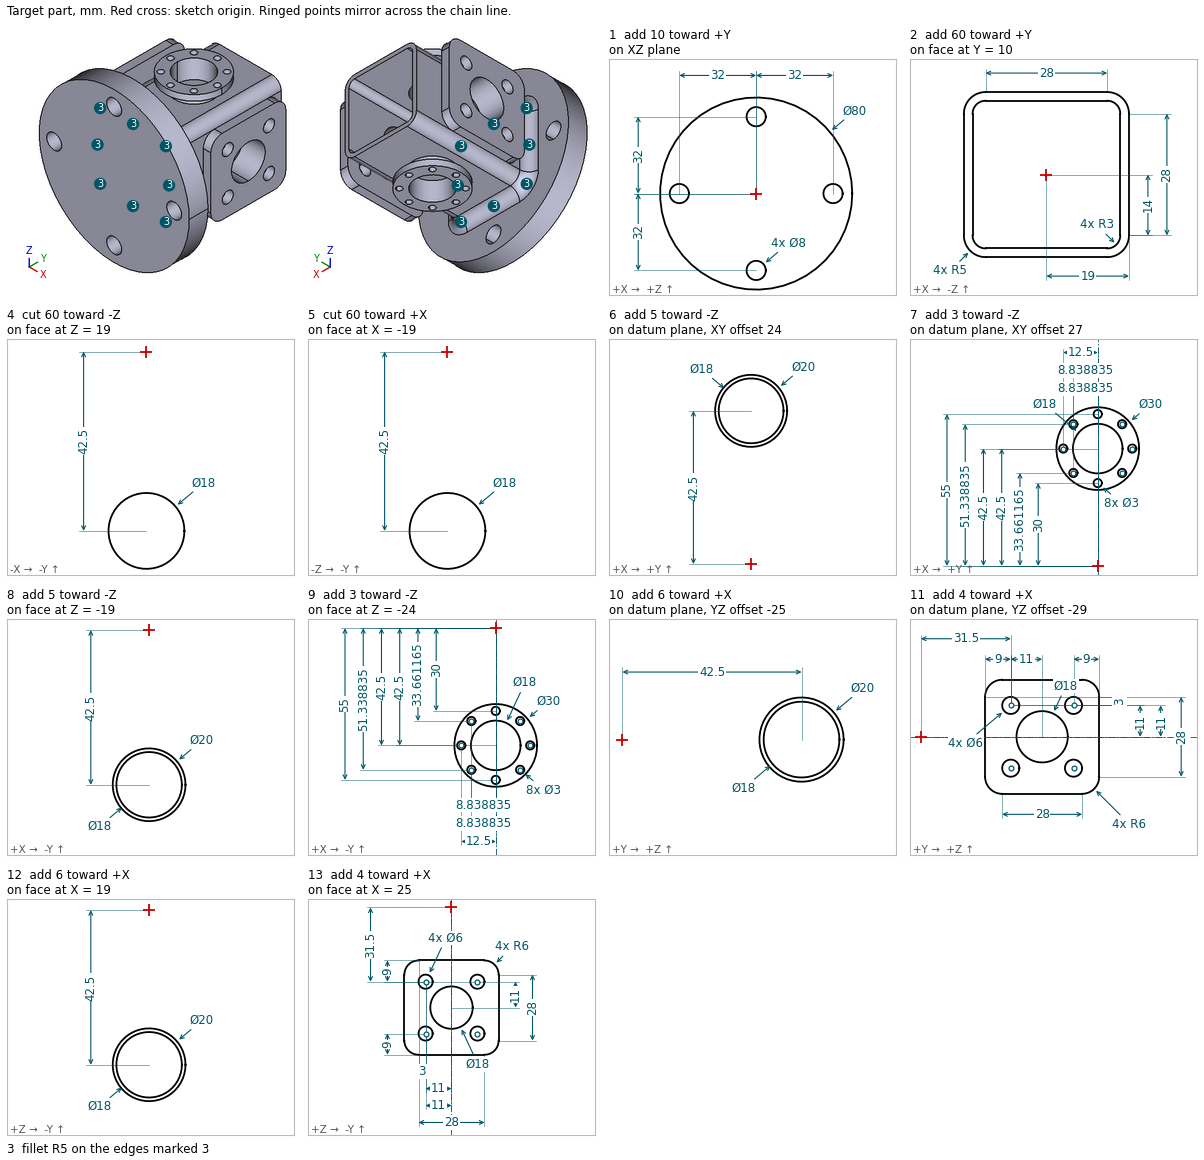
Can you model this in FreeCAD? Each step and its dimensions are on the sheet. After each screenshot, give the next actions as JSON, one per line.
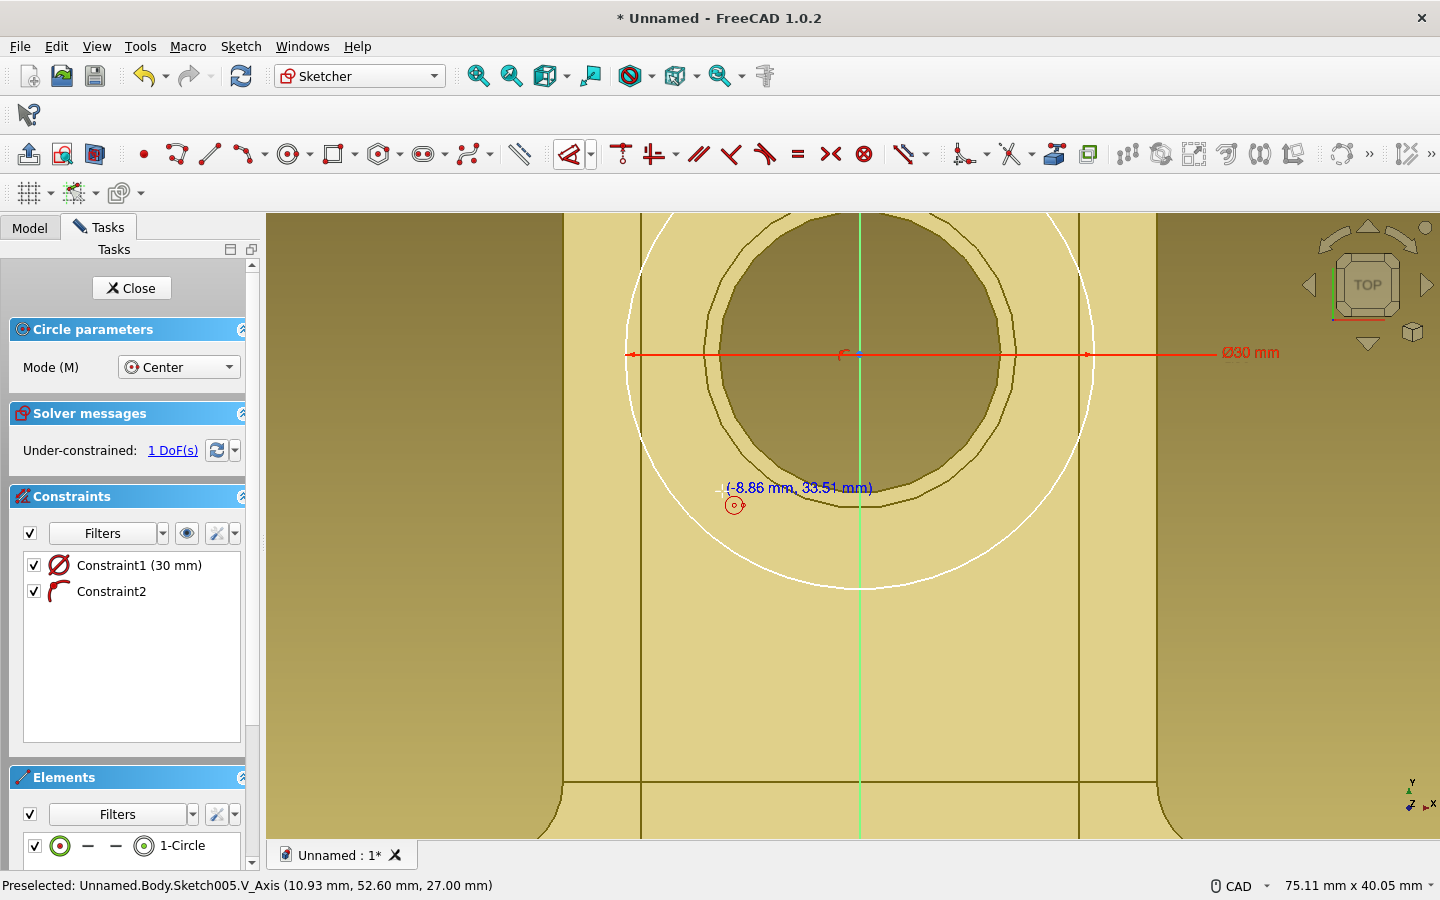
{"action": "left_click", "coordinate": [722, 490]}
{"action": "mouse_move", "coordinate": [738, 474]}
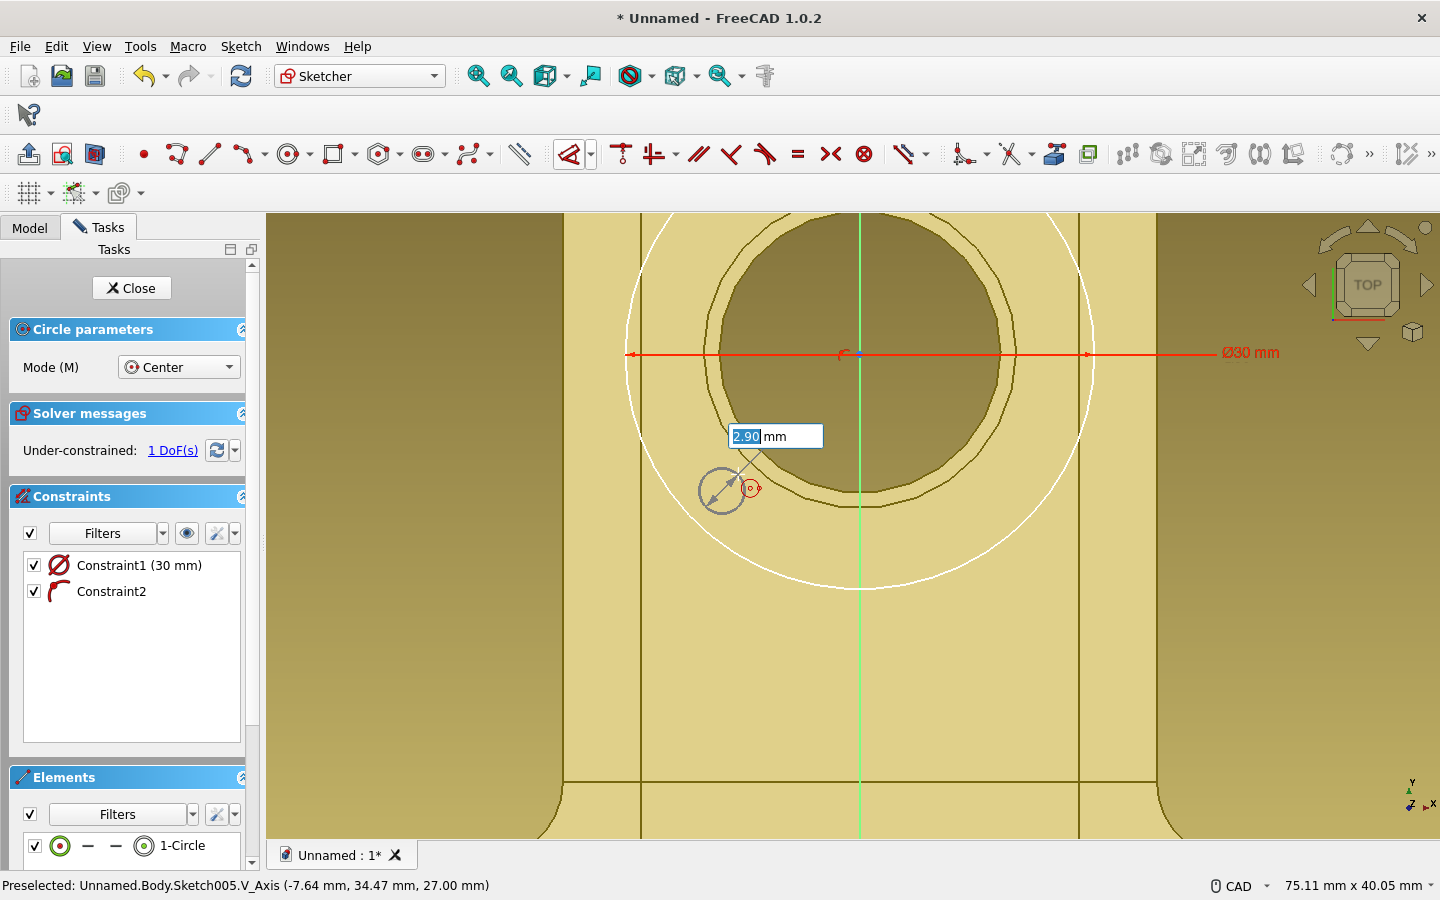
{"action": "type", "text": "3"}
{"action": "key", "text": "Return"}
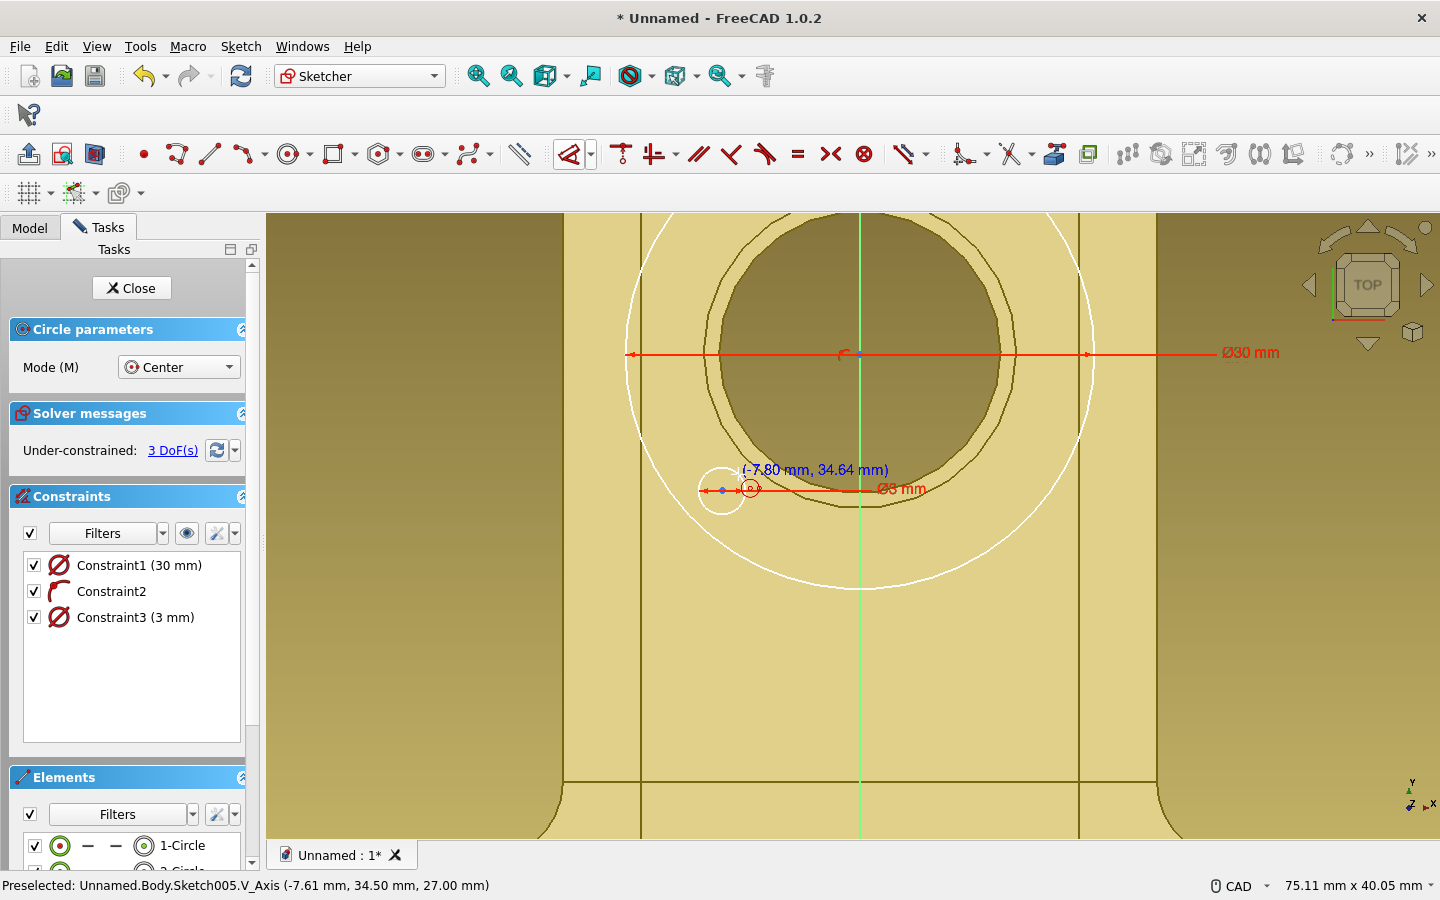
{"action": "left_click", "coordinate": [860, 547]}
{"action": "mouse_move", "coordinate": [877, 531]}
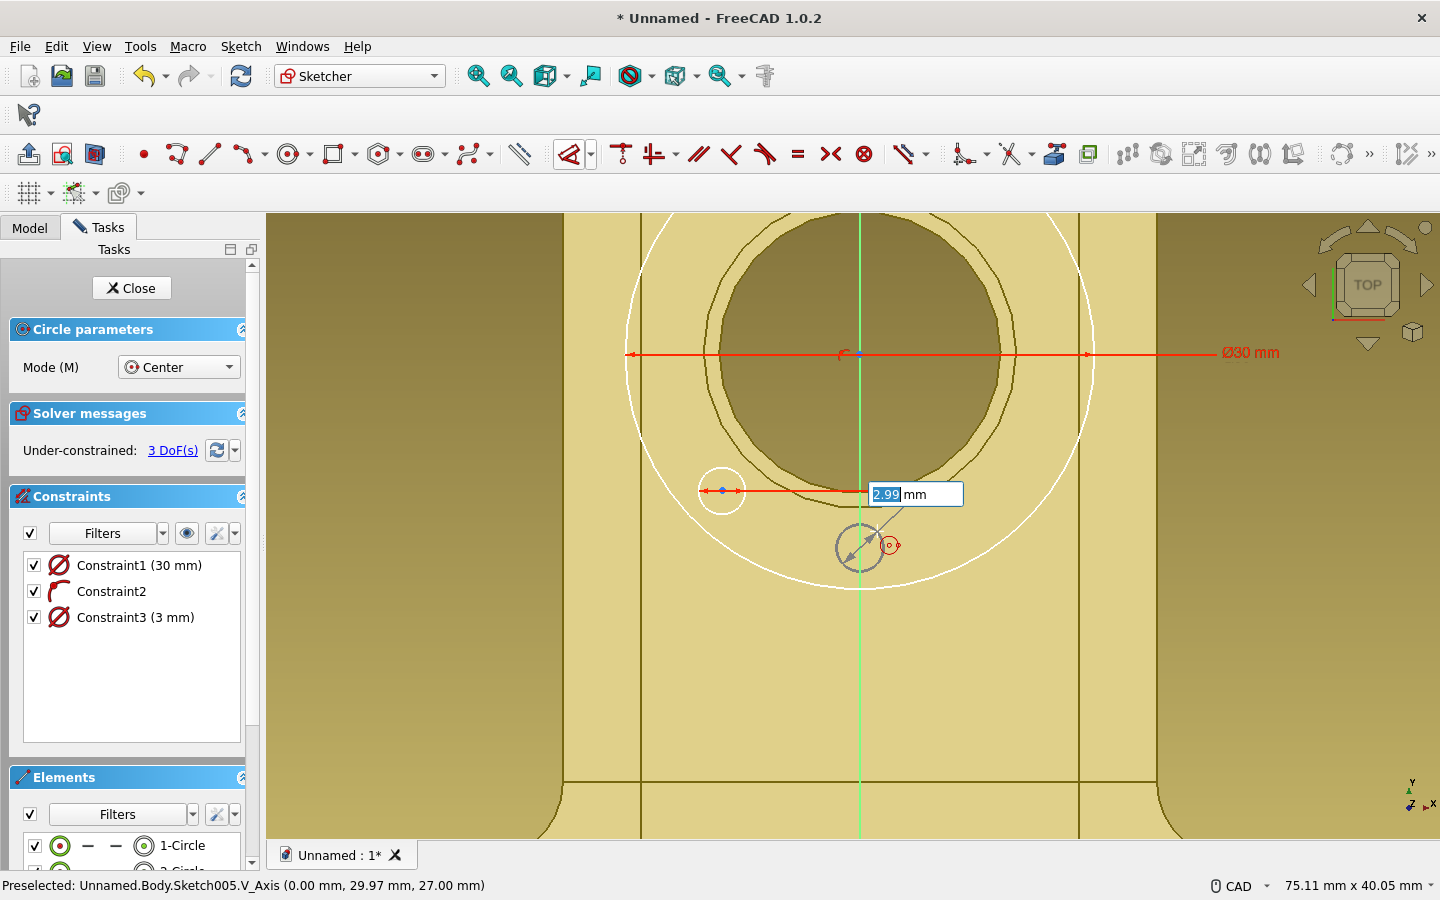
{"action": "type", "text": "3"}
{"action": "key", "text": "Return"}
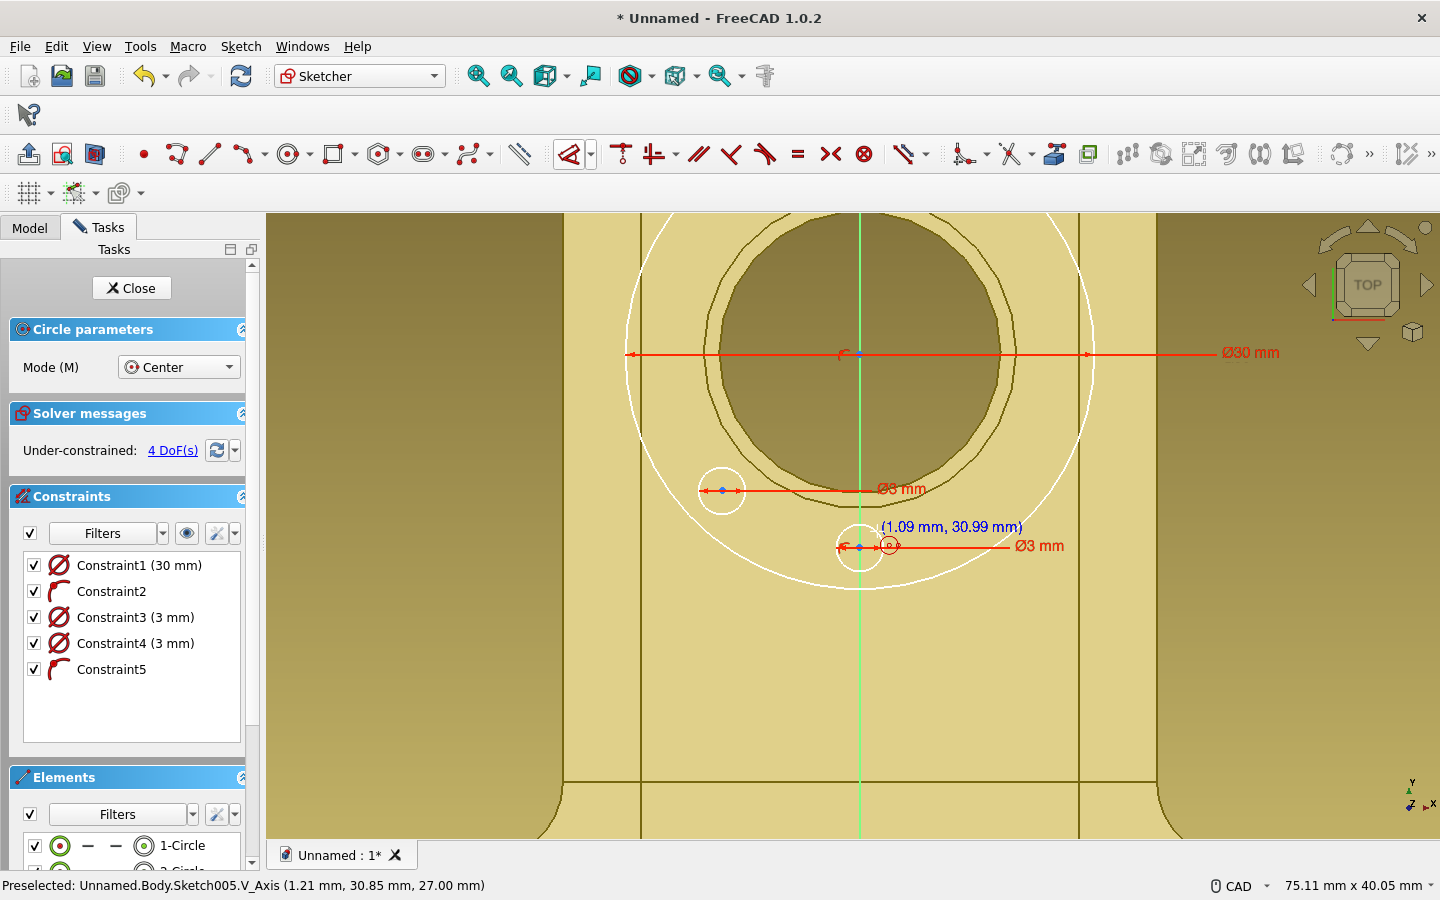
{"action": "left_click", "coordinate": [998, 490]}
{"action": "mouse_move", "coordinate": [1015, 474]}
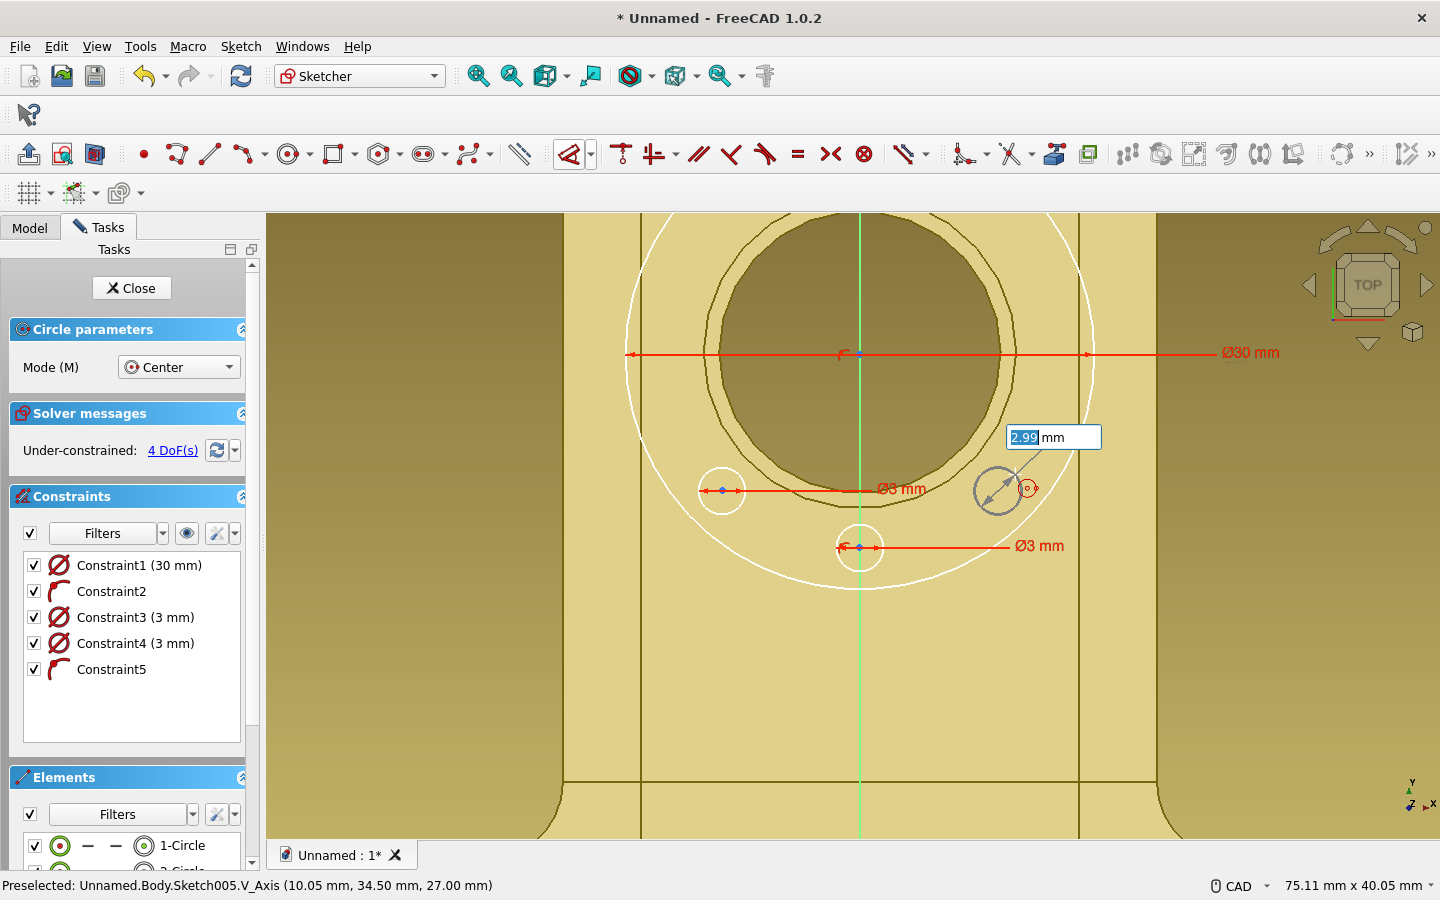
{"action": "type", "text": "3"}
{"action": "key", "text": "Return"}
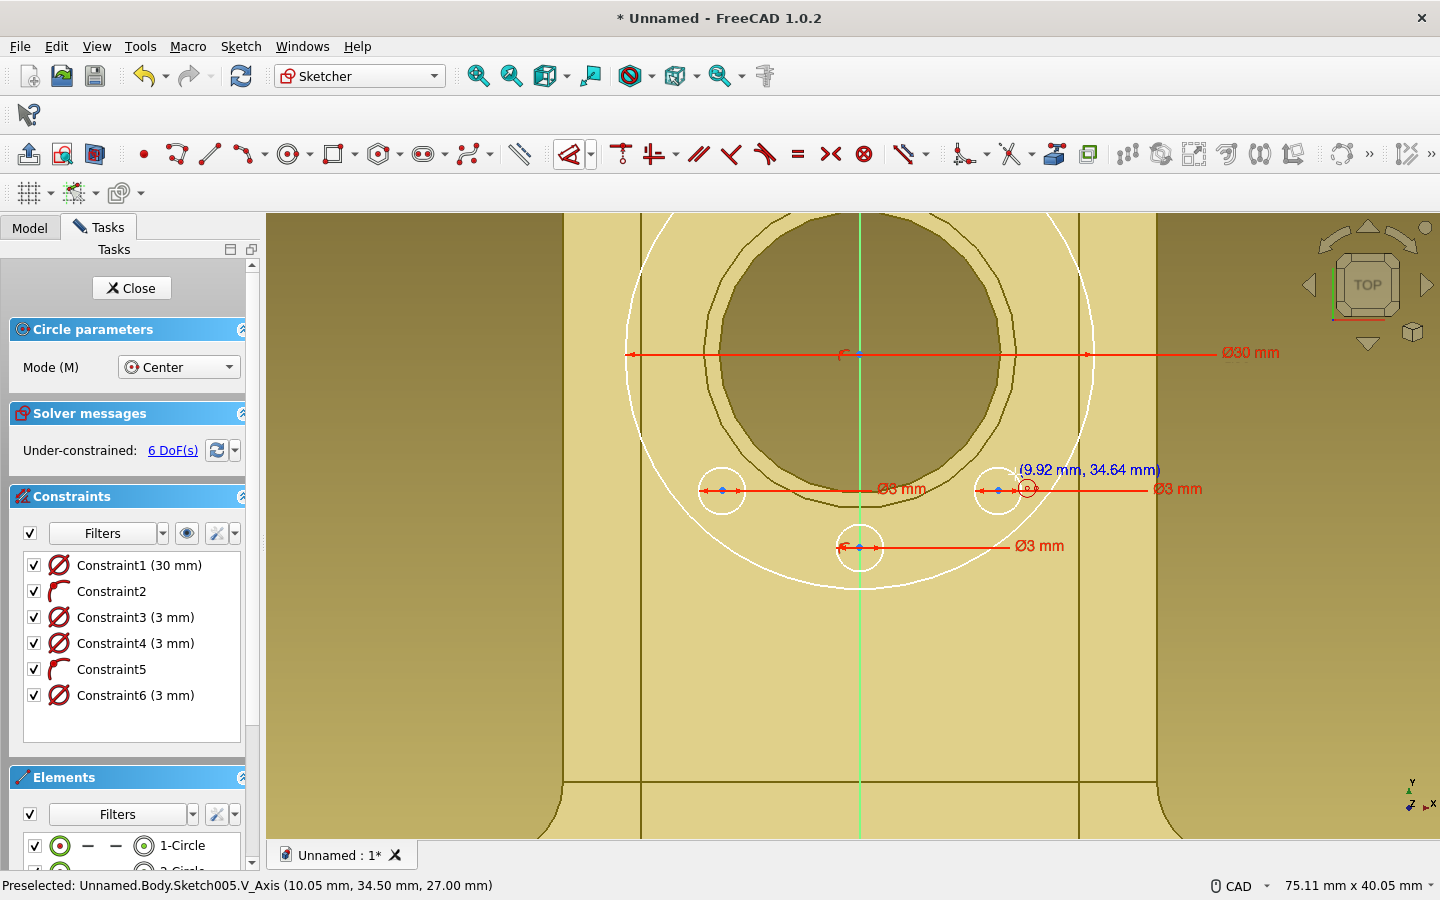
{"action": "left_click", "coordinate": [665, 352]}
{"action": "mouse_move", "coordinate": [681, 336]}